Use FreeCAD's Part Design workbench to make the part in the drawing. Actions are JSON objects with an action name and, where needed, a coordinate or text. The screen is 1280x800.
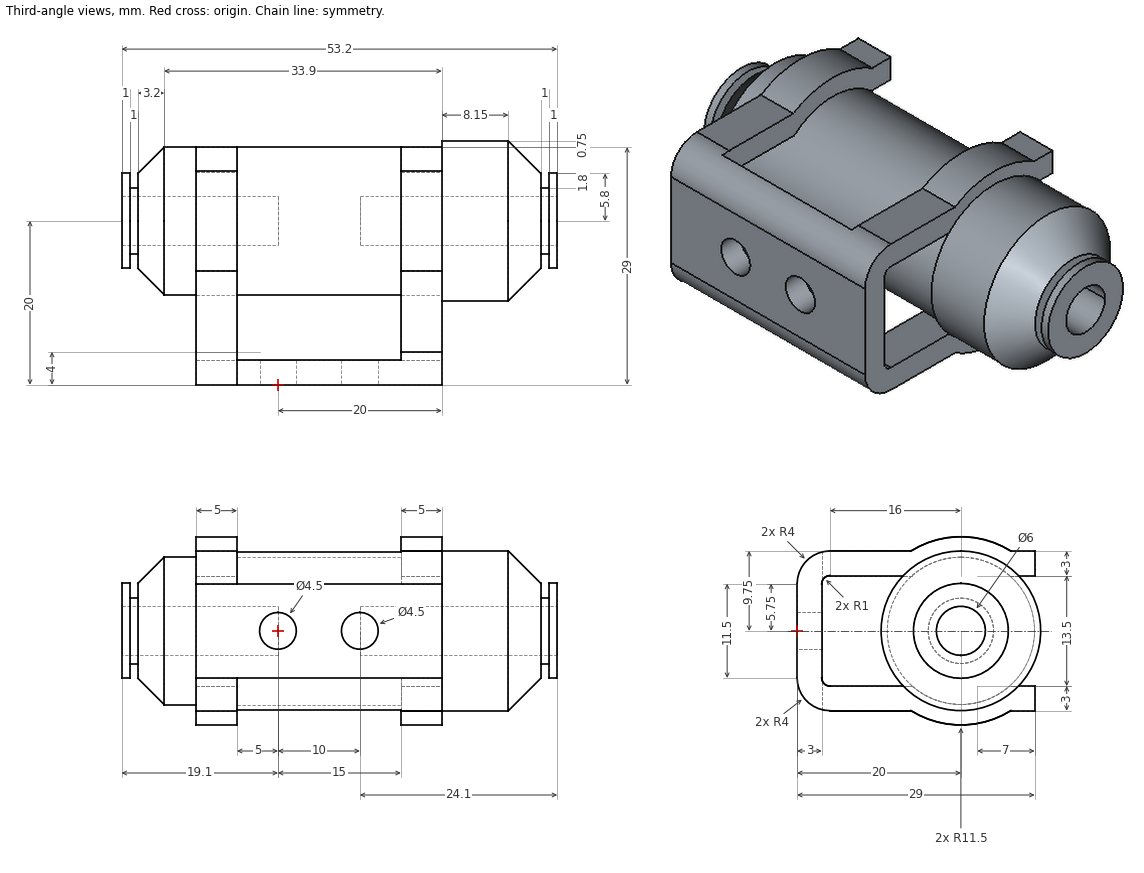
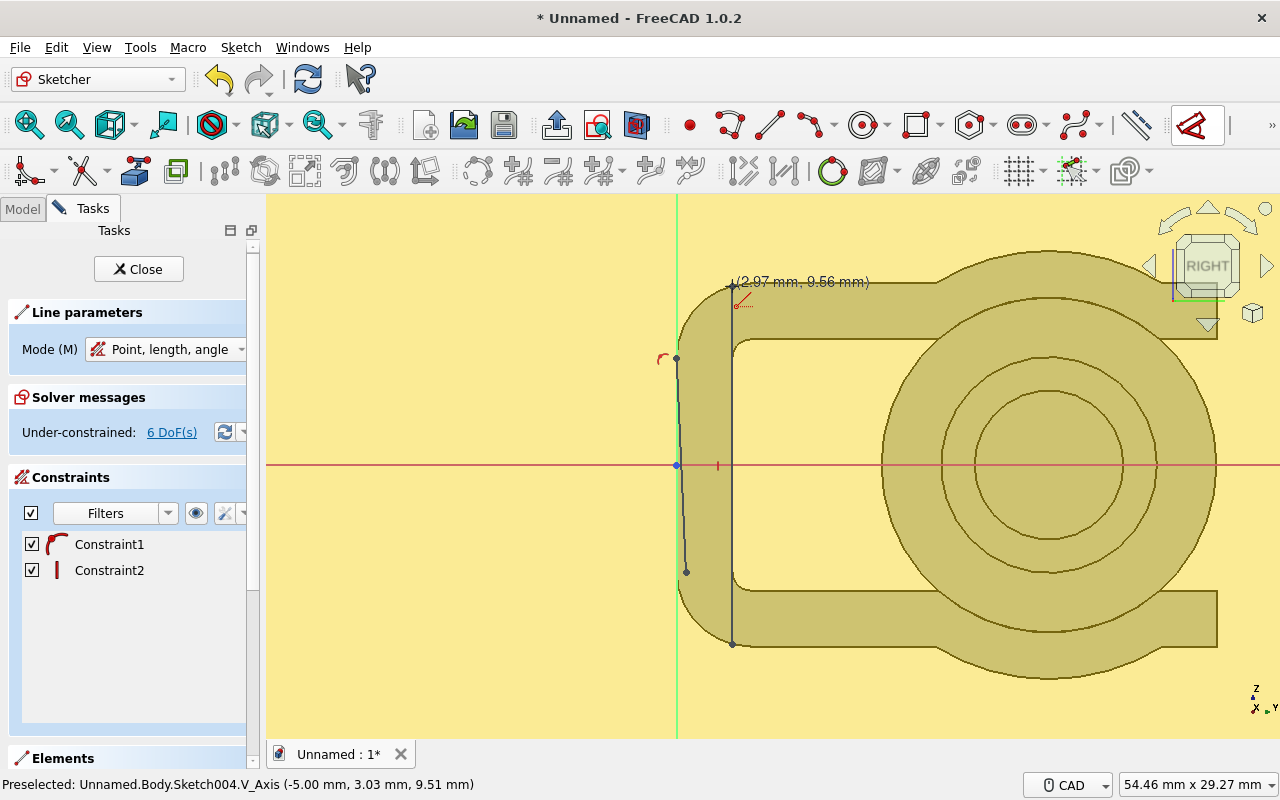
{"action": "left_click", "coordinate": [810, 126]}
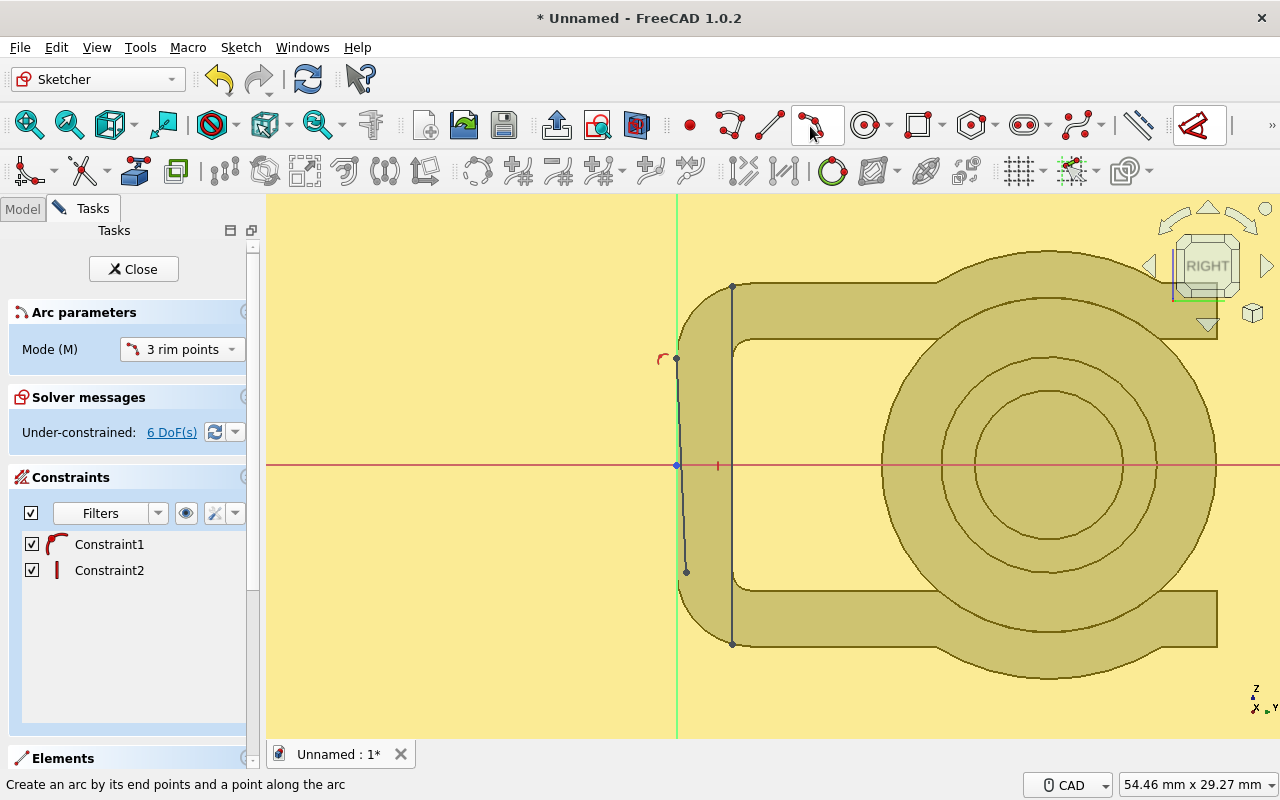
{"action": "left_click", "coordinate": [686, 573]}
{"action": "left_click", "coordinate": [732, 645]}
{"action": "left_click", "coordinate": [692, 618]}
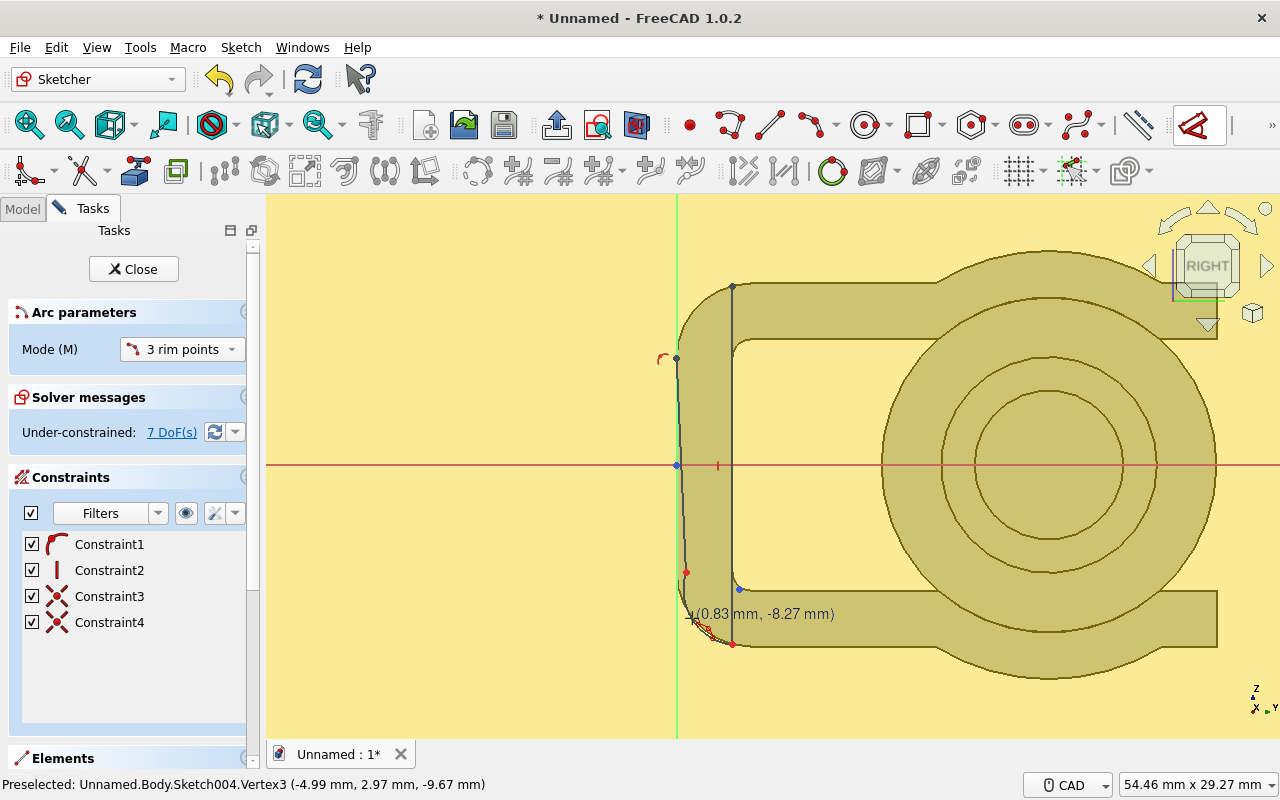
{"action": "left_click", "coordinate": [732, 287]}
{"action": "left_click", "coordinate": [677, 359]}
{"action": "left_click", "coordinate": [692, 312]}
{"action": "key", "text": "Escape"}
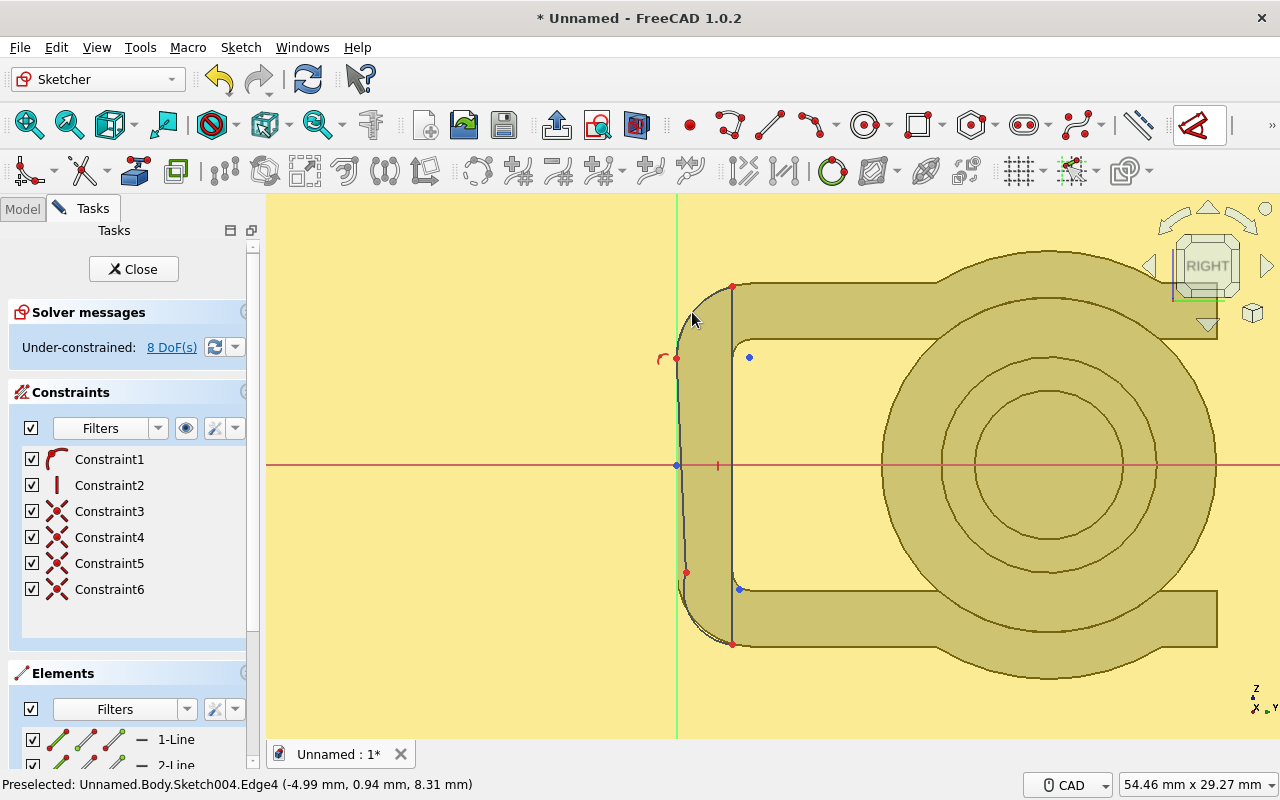
{"action": "left_click", "coordinate": [679, 423]}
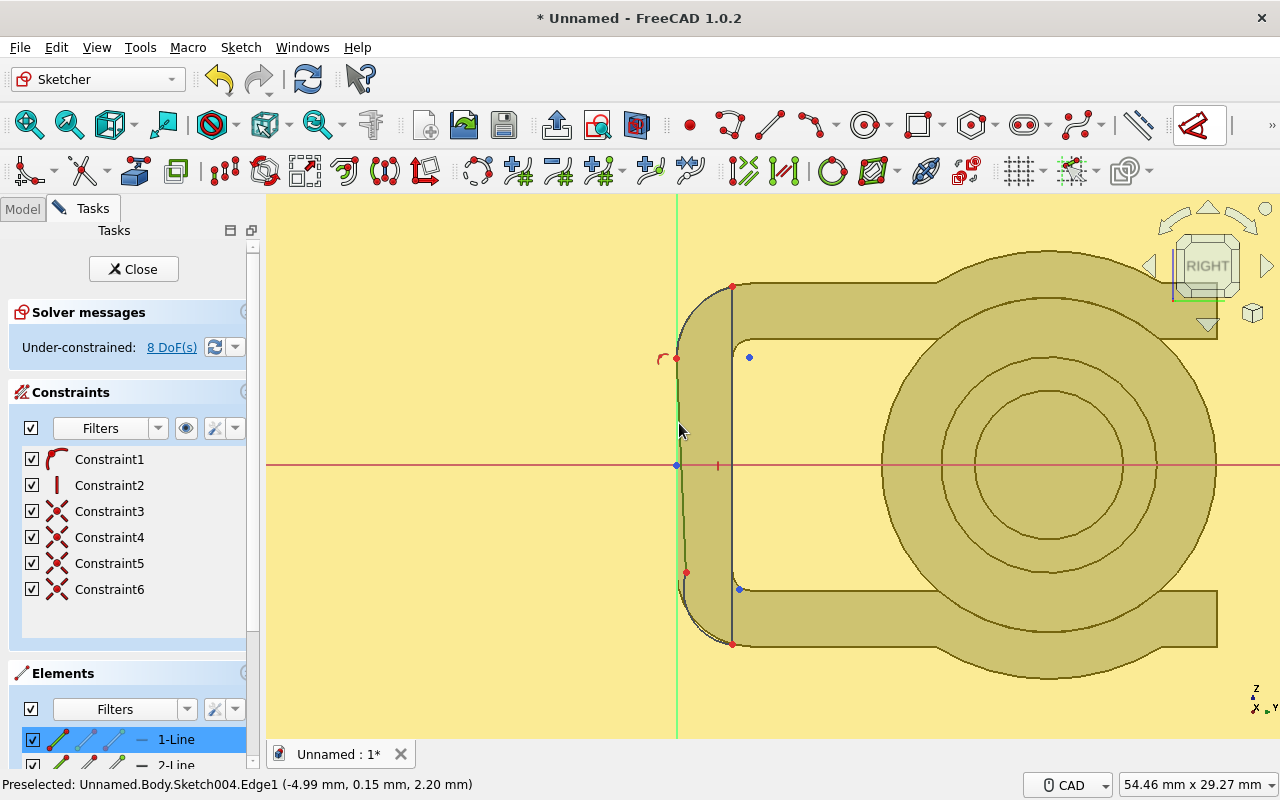
{"action": "left_click", "coordinate": [705, 634]}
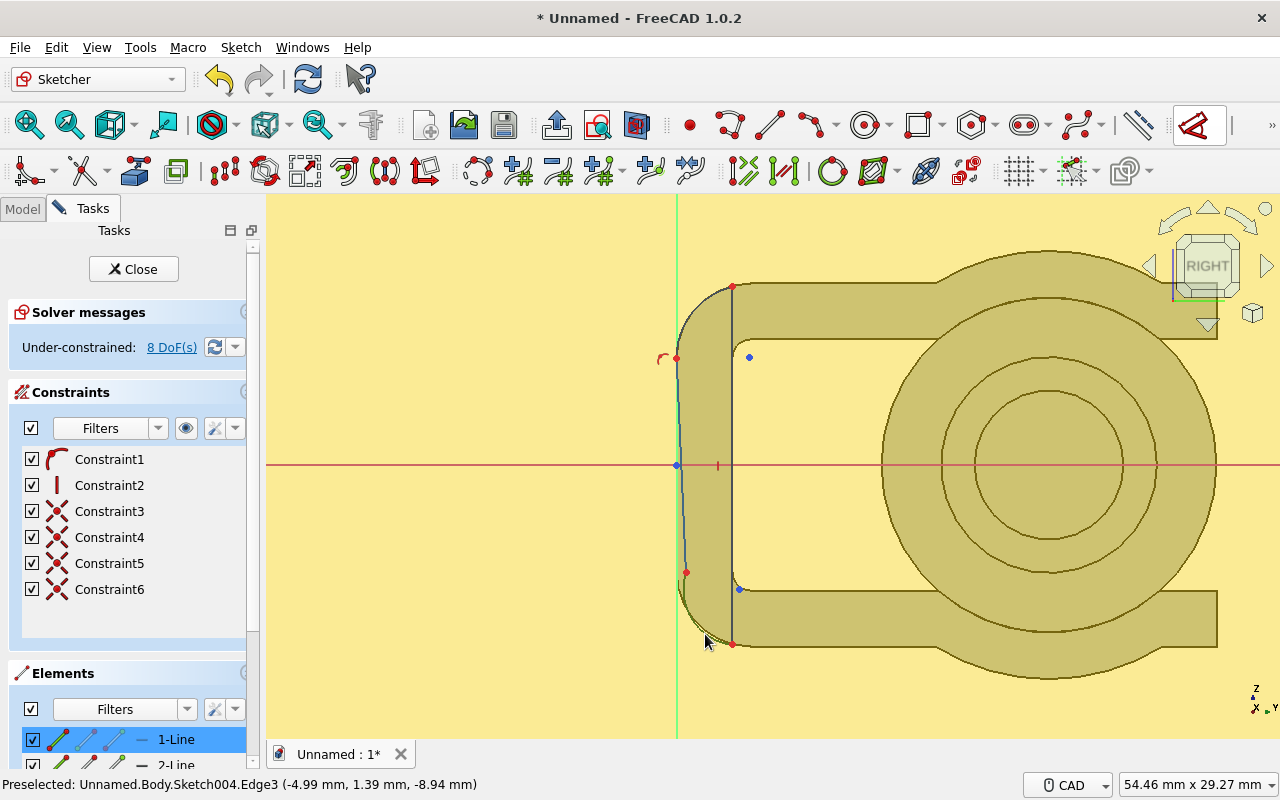
{"action": "key", "text": "t"}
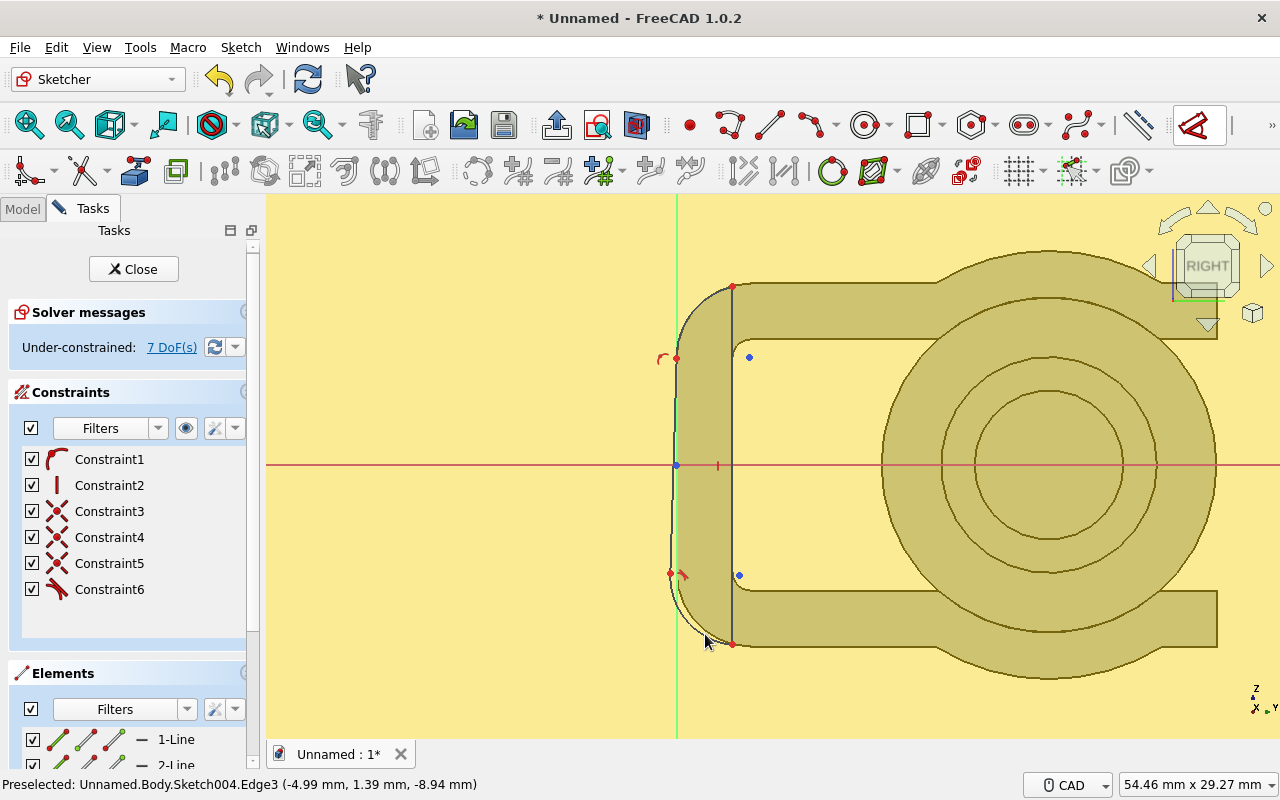
{"action": "left_click", "coordinate": [675, 423]}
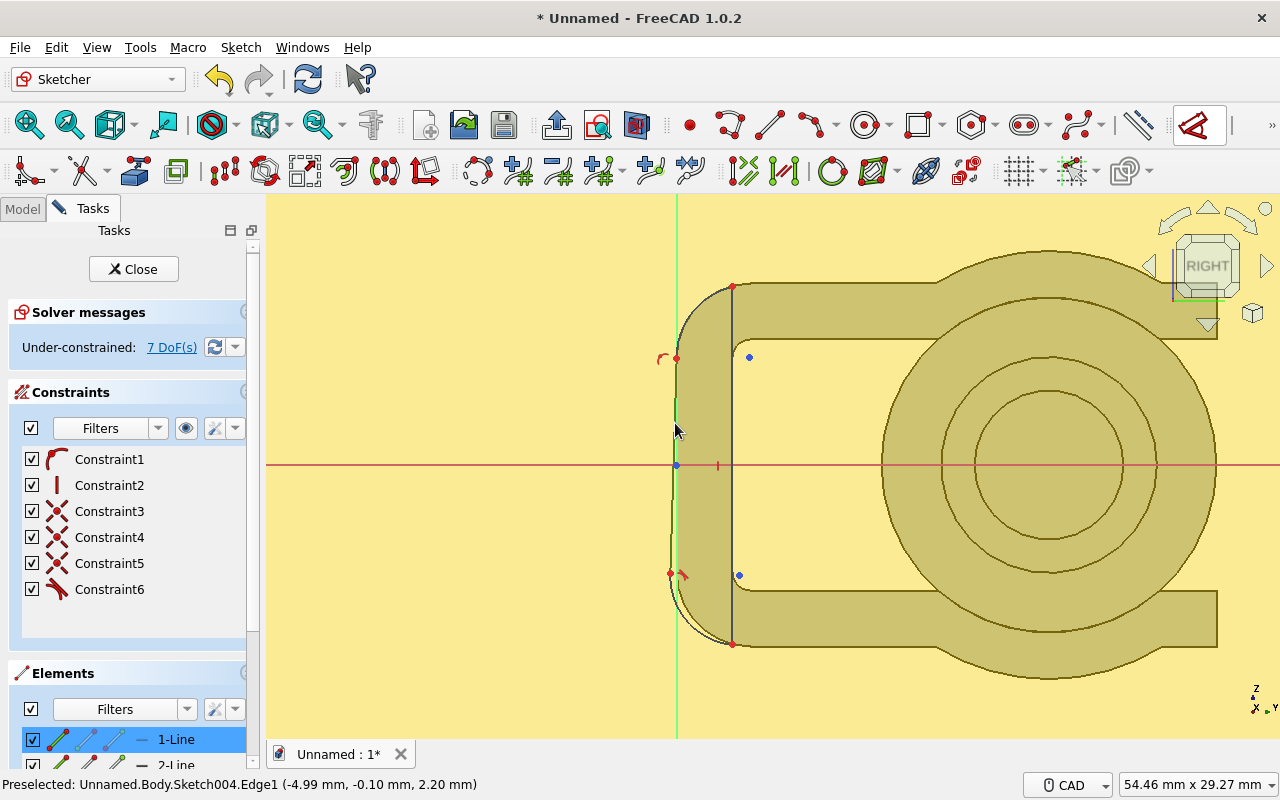
{"action": "left_click", "coordinate": [706, 300]}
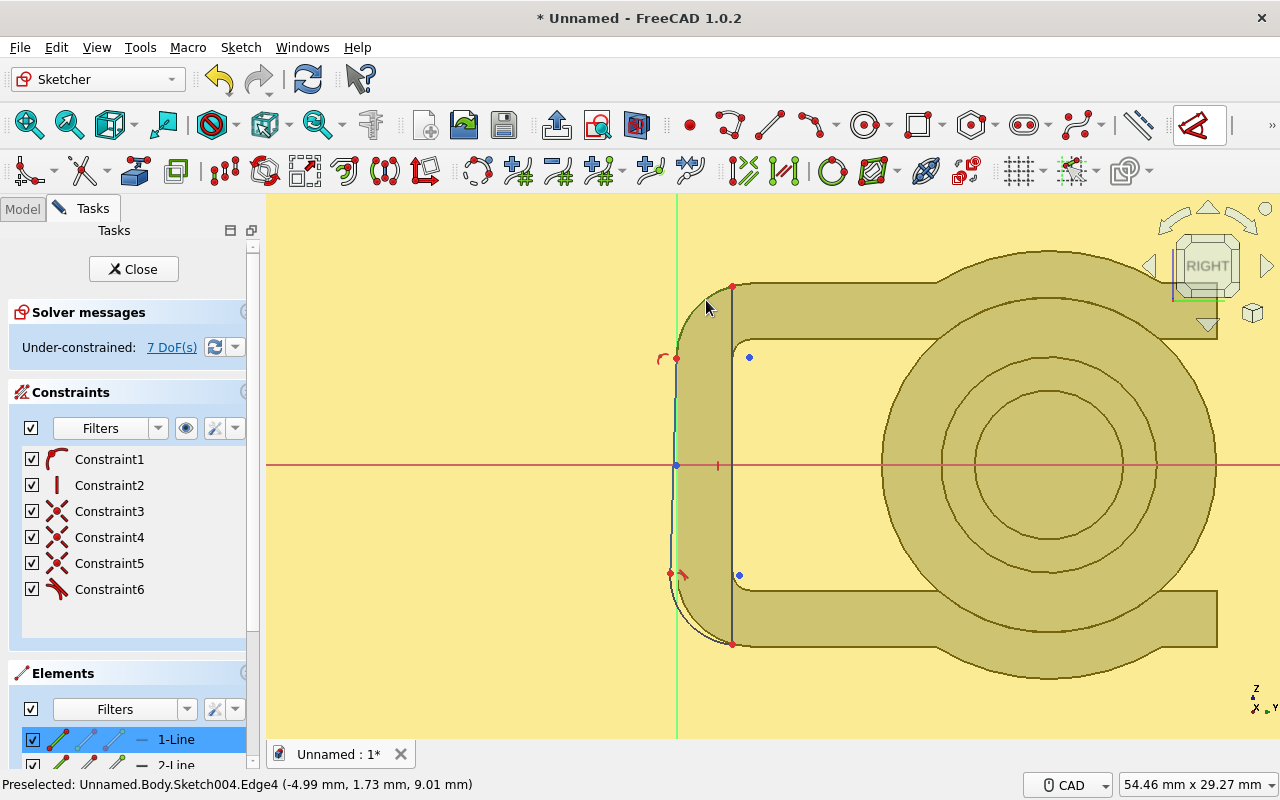
{"action": "key", "text": "t"}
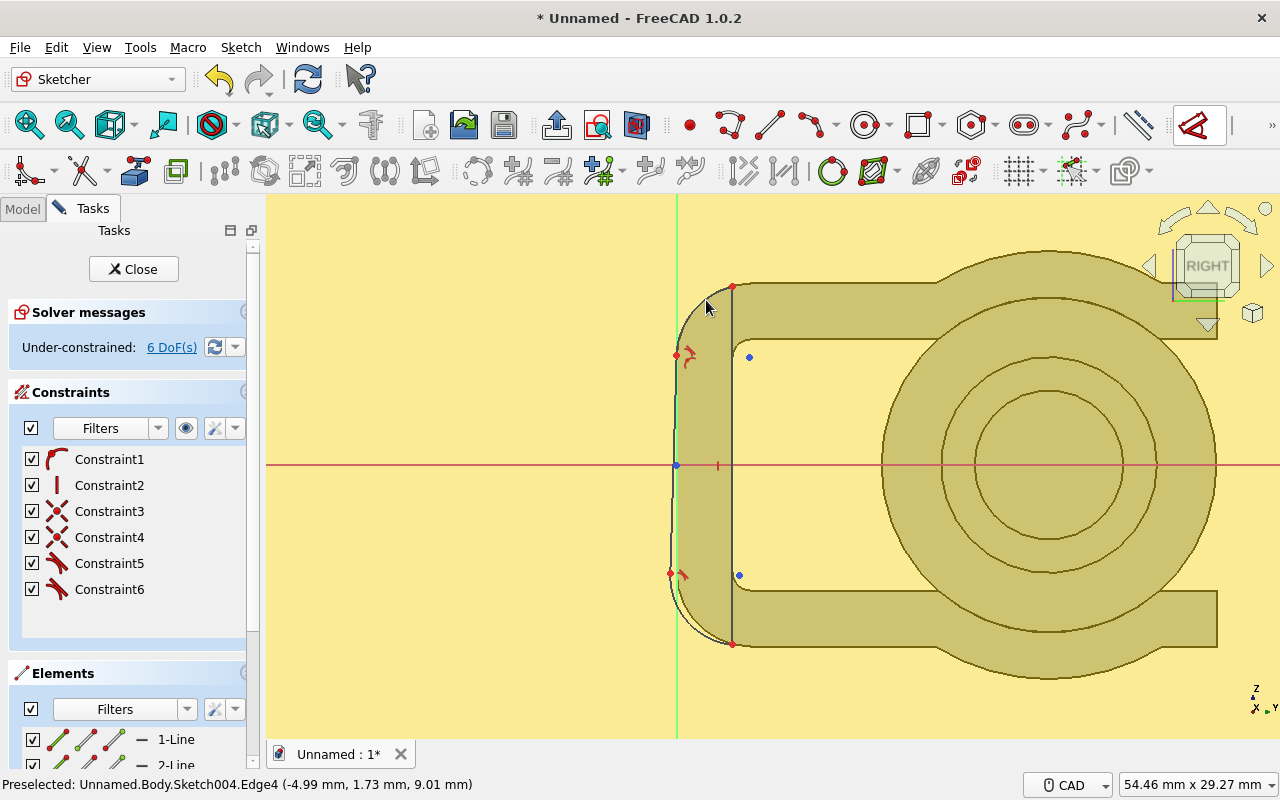
{"action": "left_click", "coordinate": [675, 421]}